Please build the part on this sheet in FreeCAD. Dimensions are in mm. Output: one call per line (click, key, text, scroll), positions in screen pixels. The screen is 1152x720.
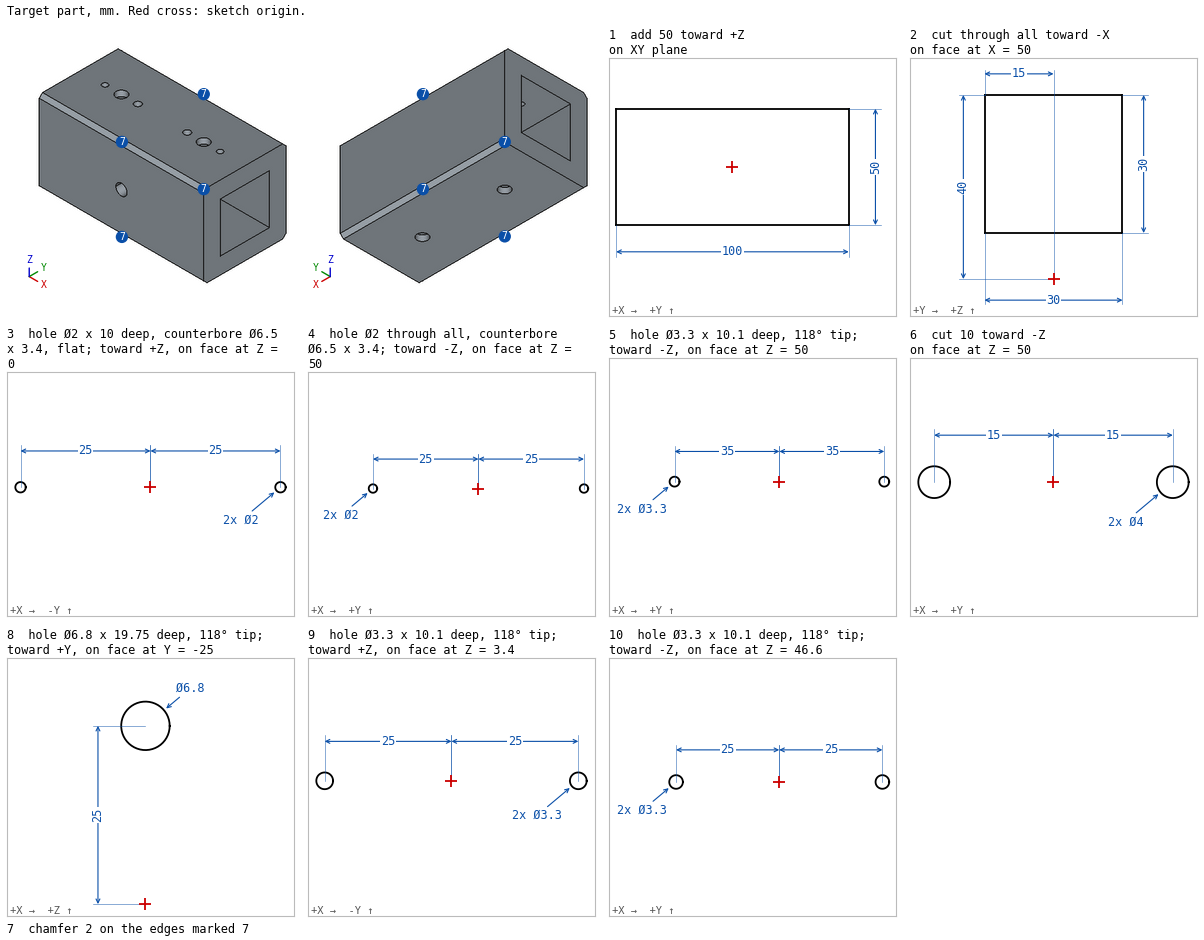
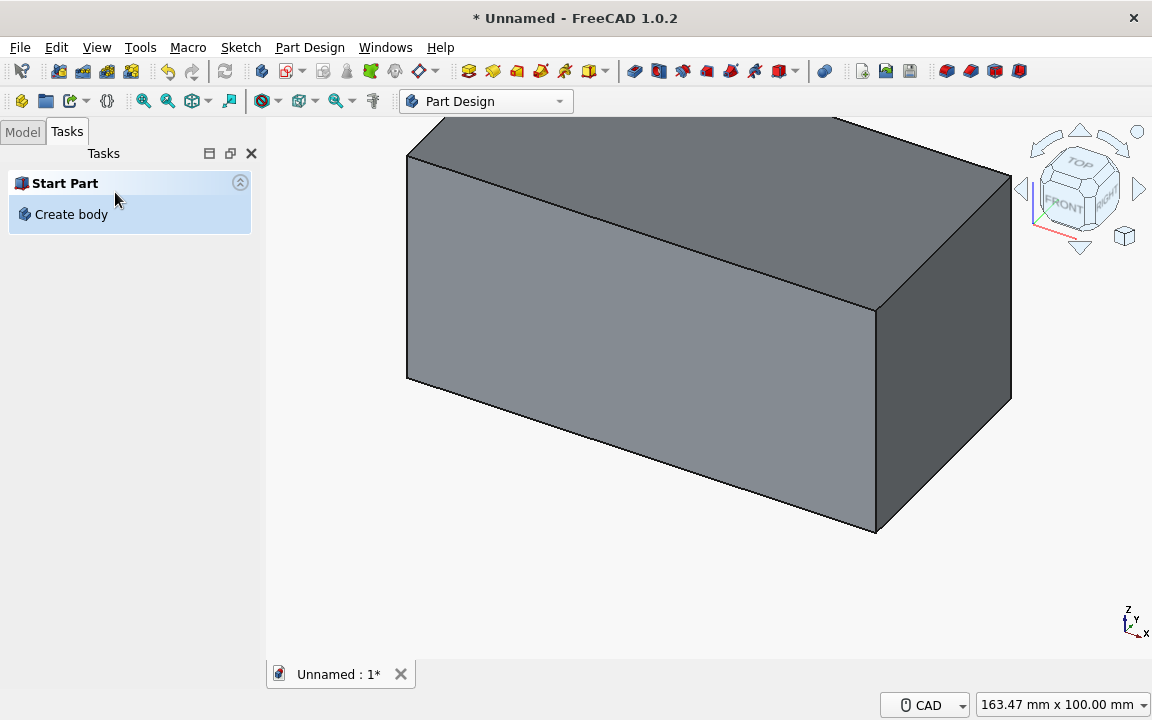
click(144, 102)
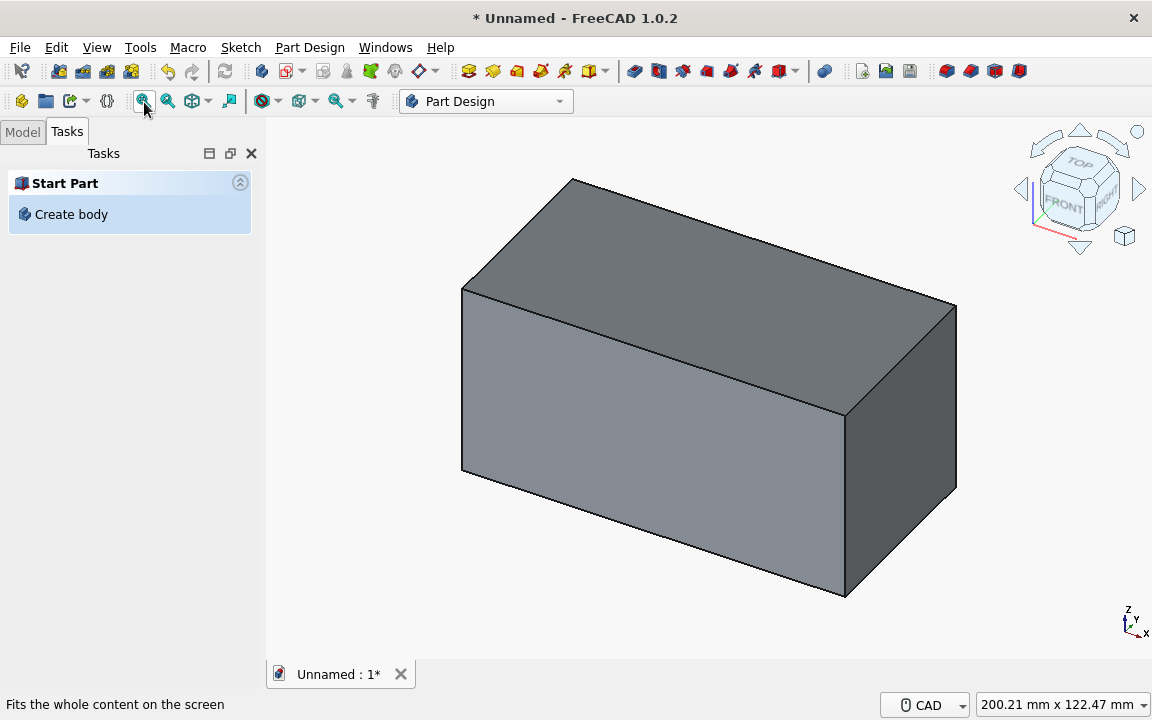
click(901, 450)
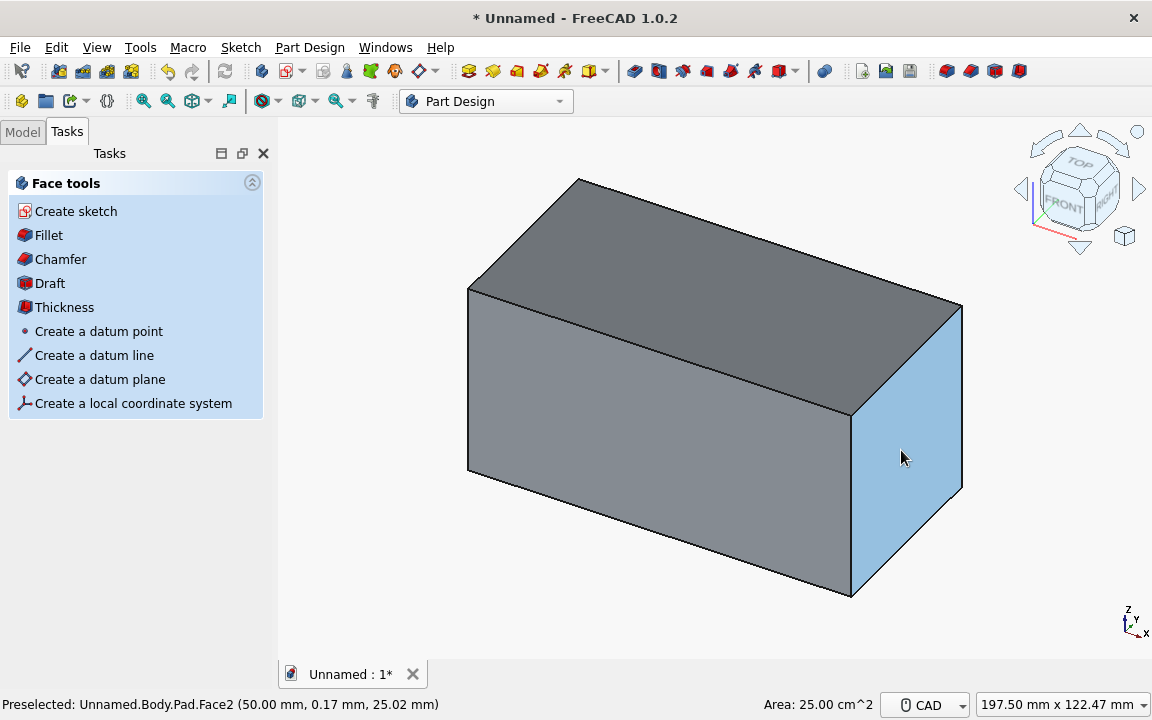
click(286, 72)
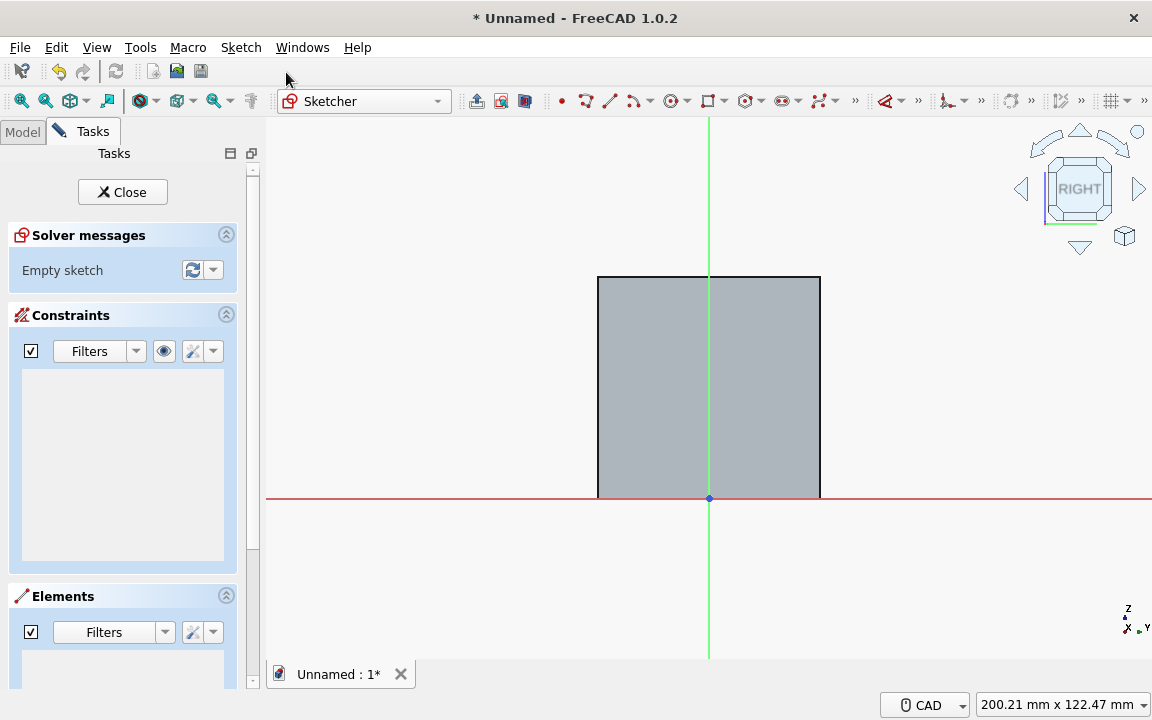
scroll(792, 437, up, 3)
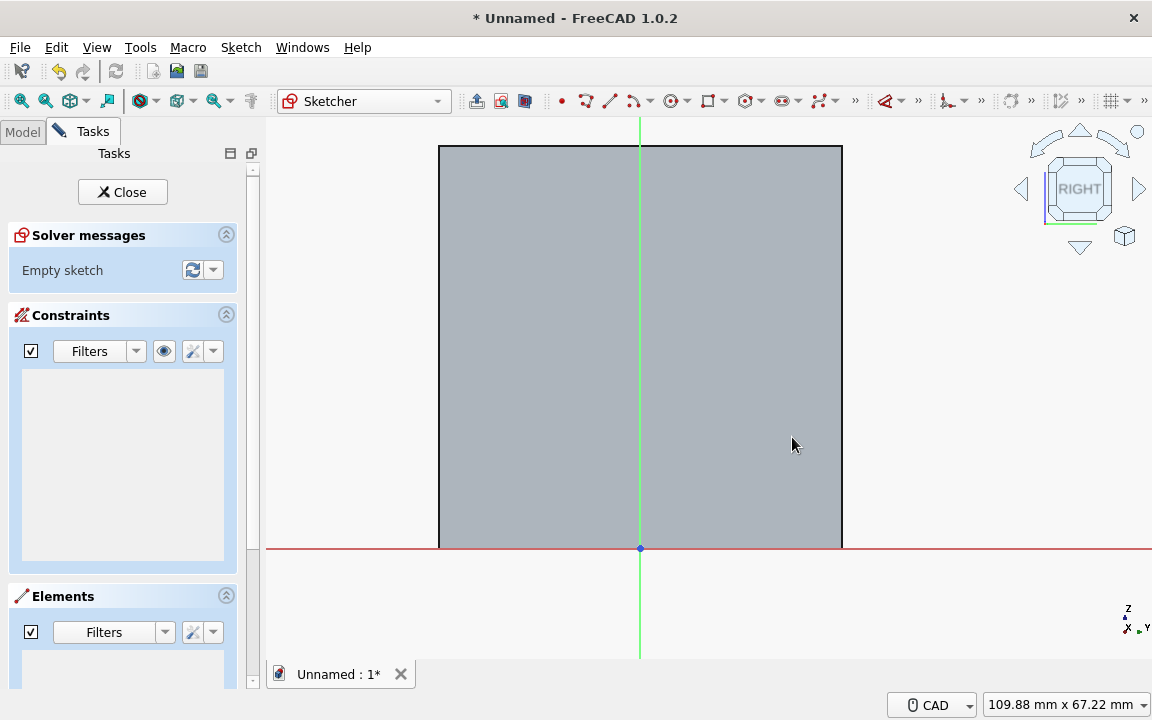
click(708, 102)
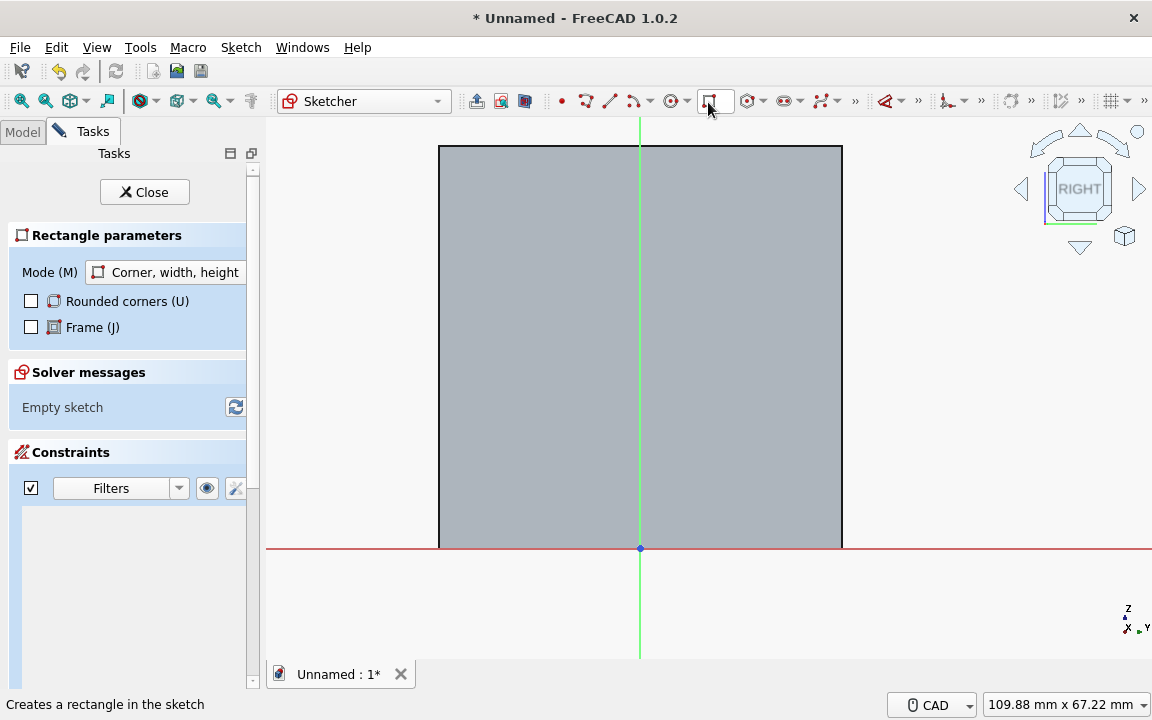
click(519, 226)
move(761, 468)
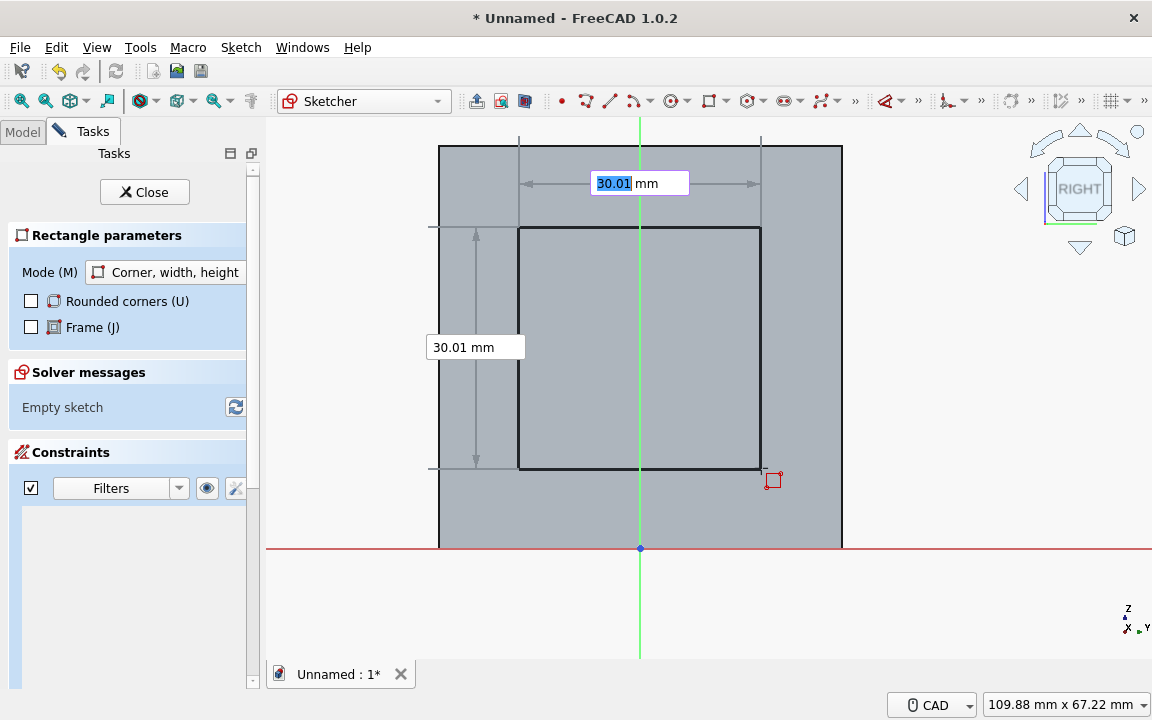
text(30)
key(Tab)
text(30)
key(Return)
key(Escape)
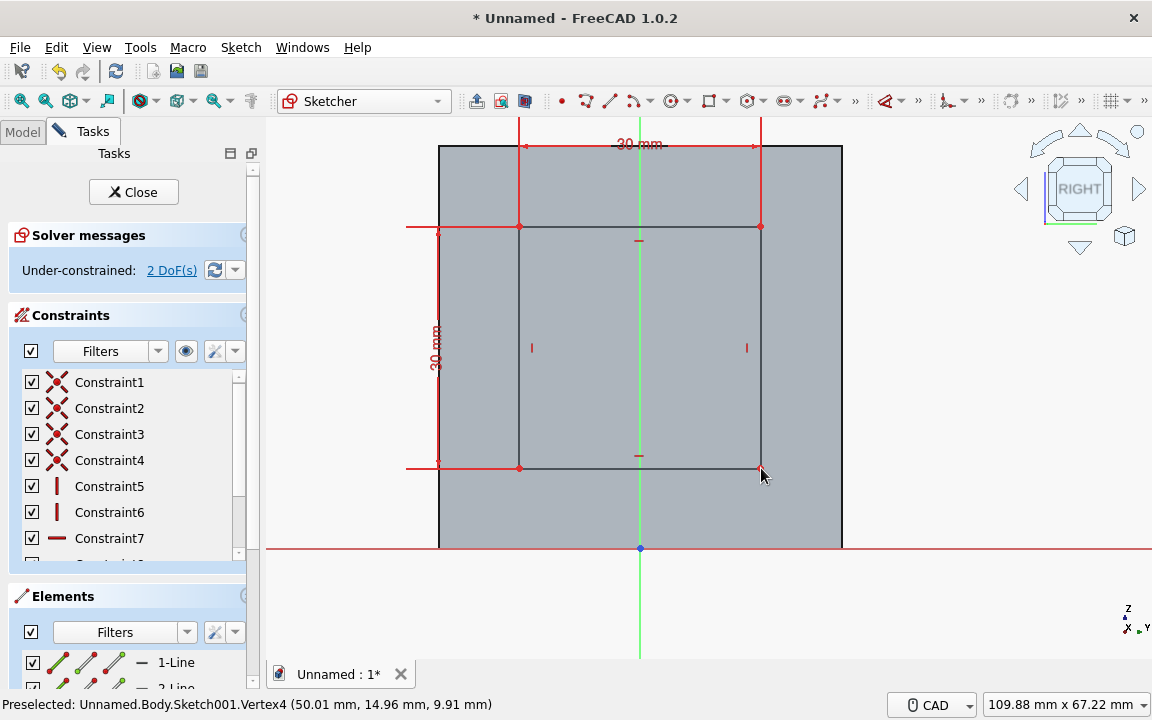
click(519, 227)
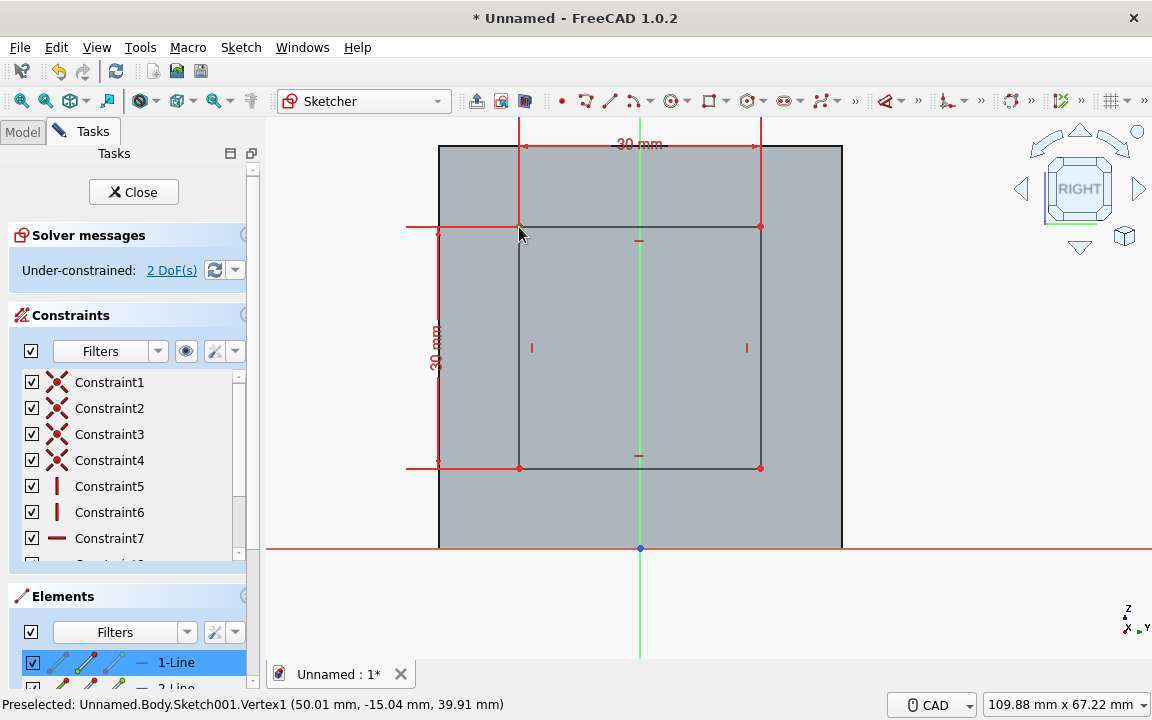
click(904, 102)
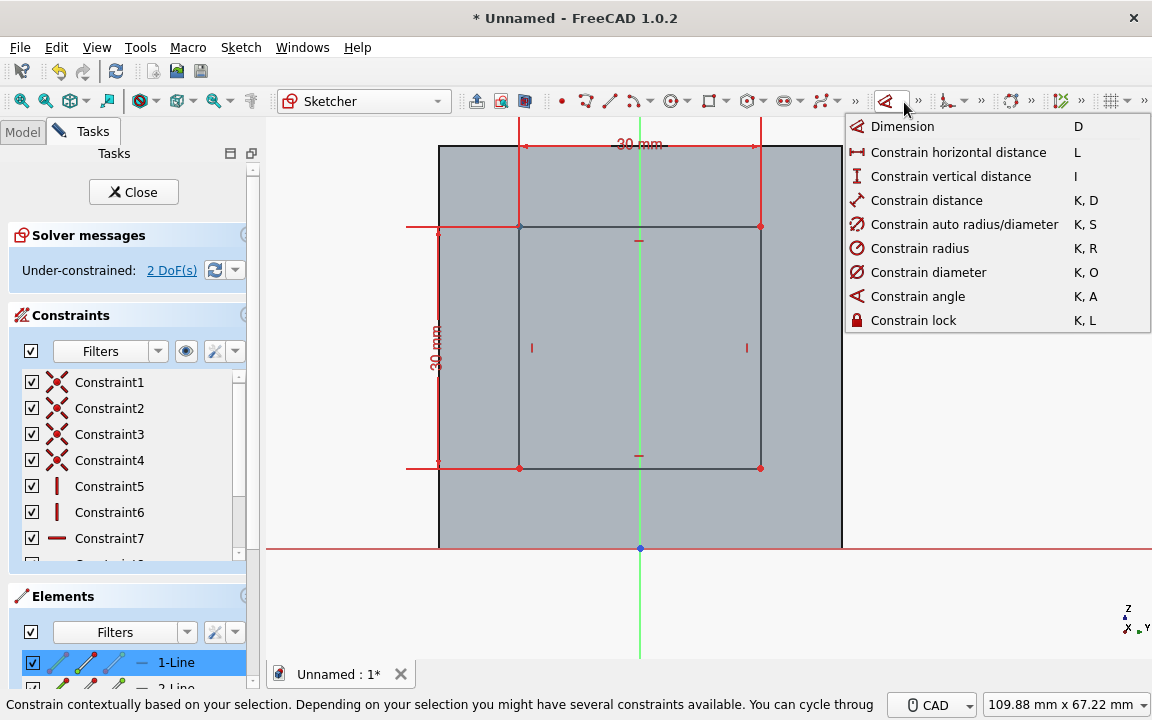
click(998, 152)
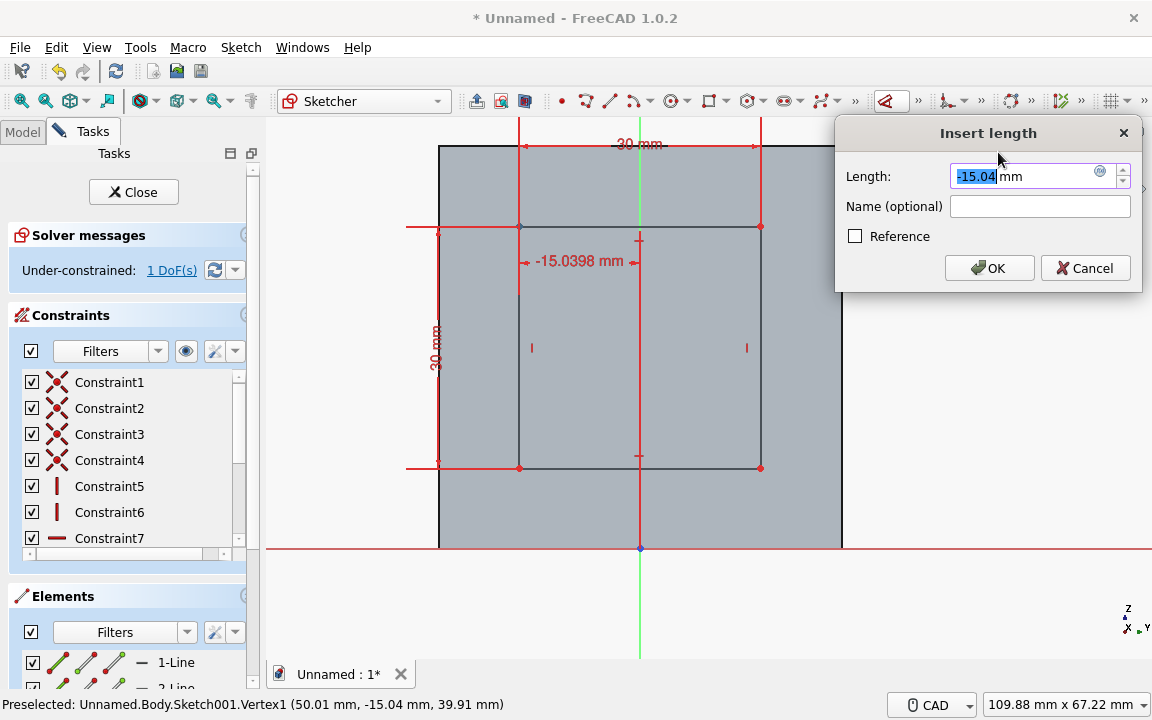
text(-15)
key(Return)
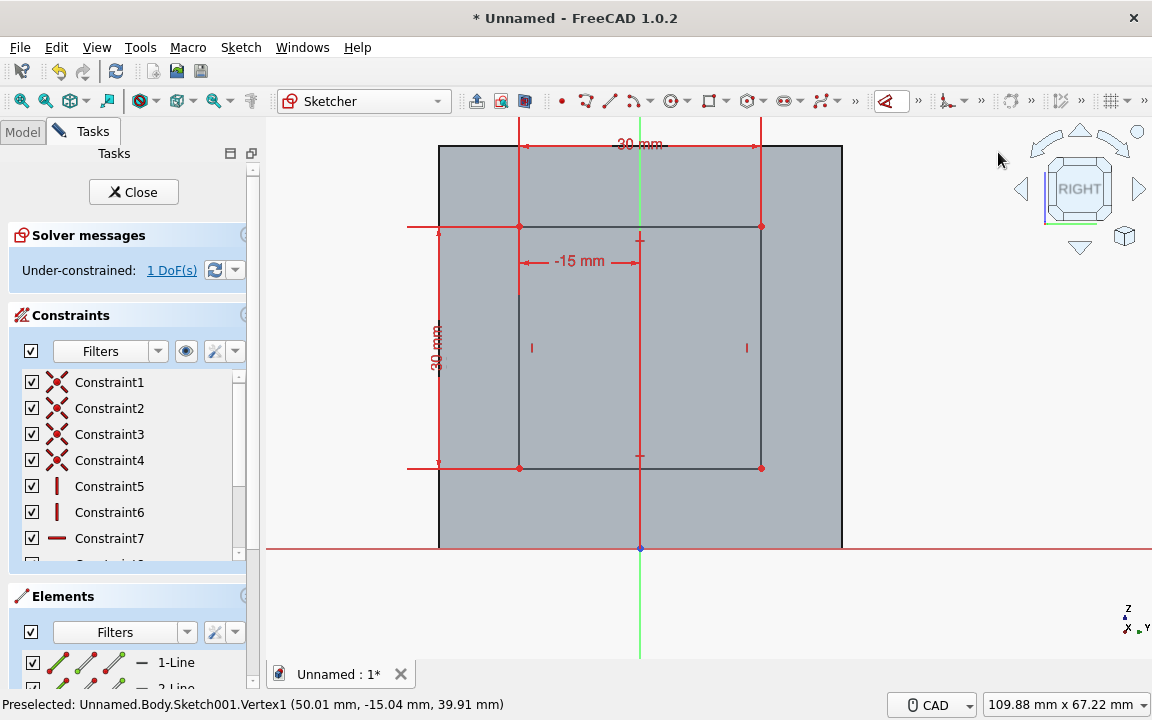
click(519, 227)